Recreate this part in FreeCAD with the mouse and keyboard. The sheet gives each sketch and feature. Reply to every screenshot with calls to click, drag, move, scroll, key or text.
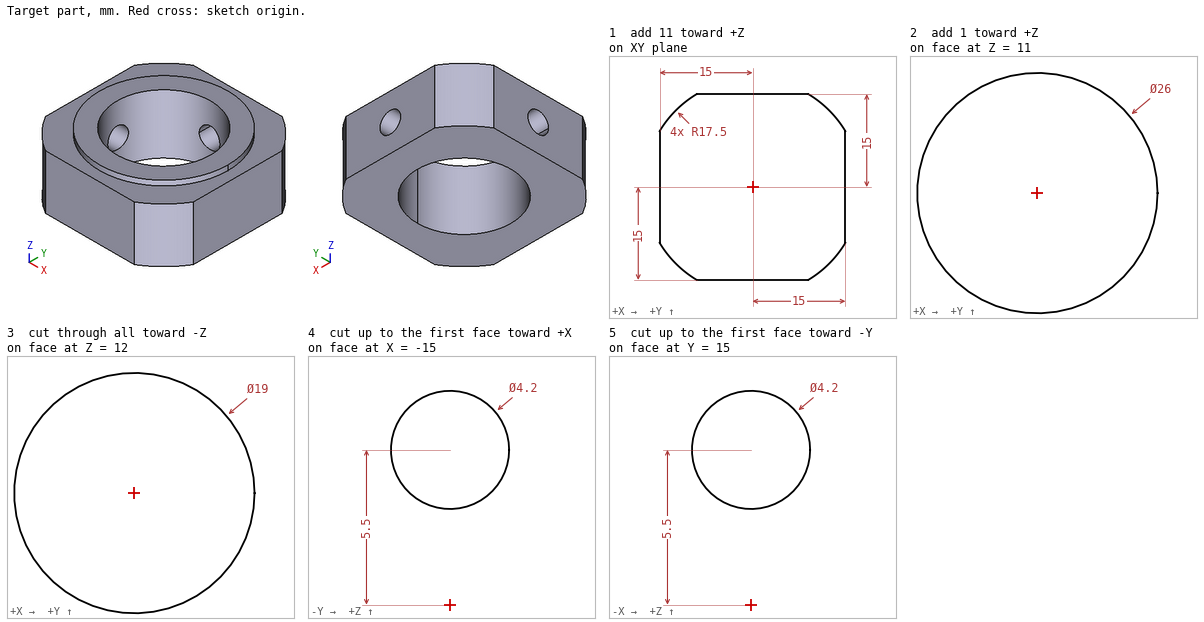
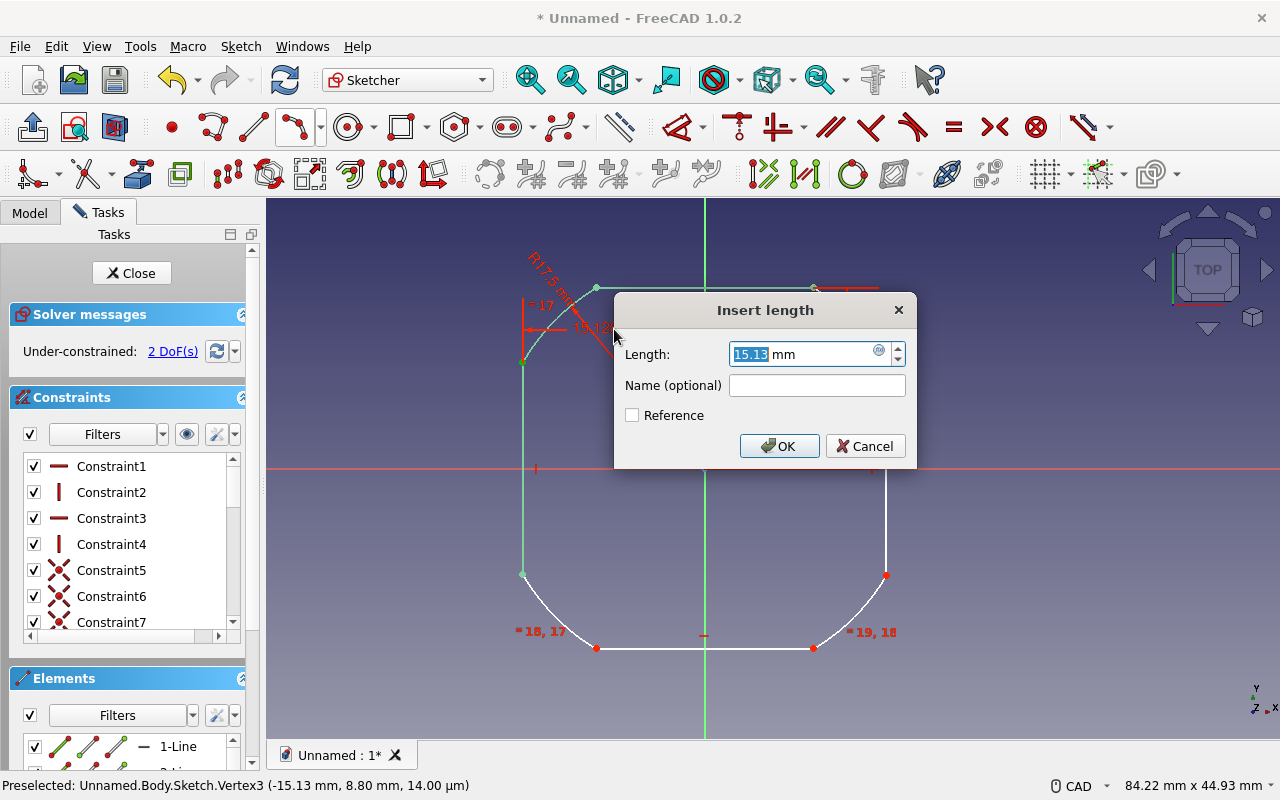
text(15)
key(Return)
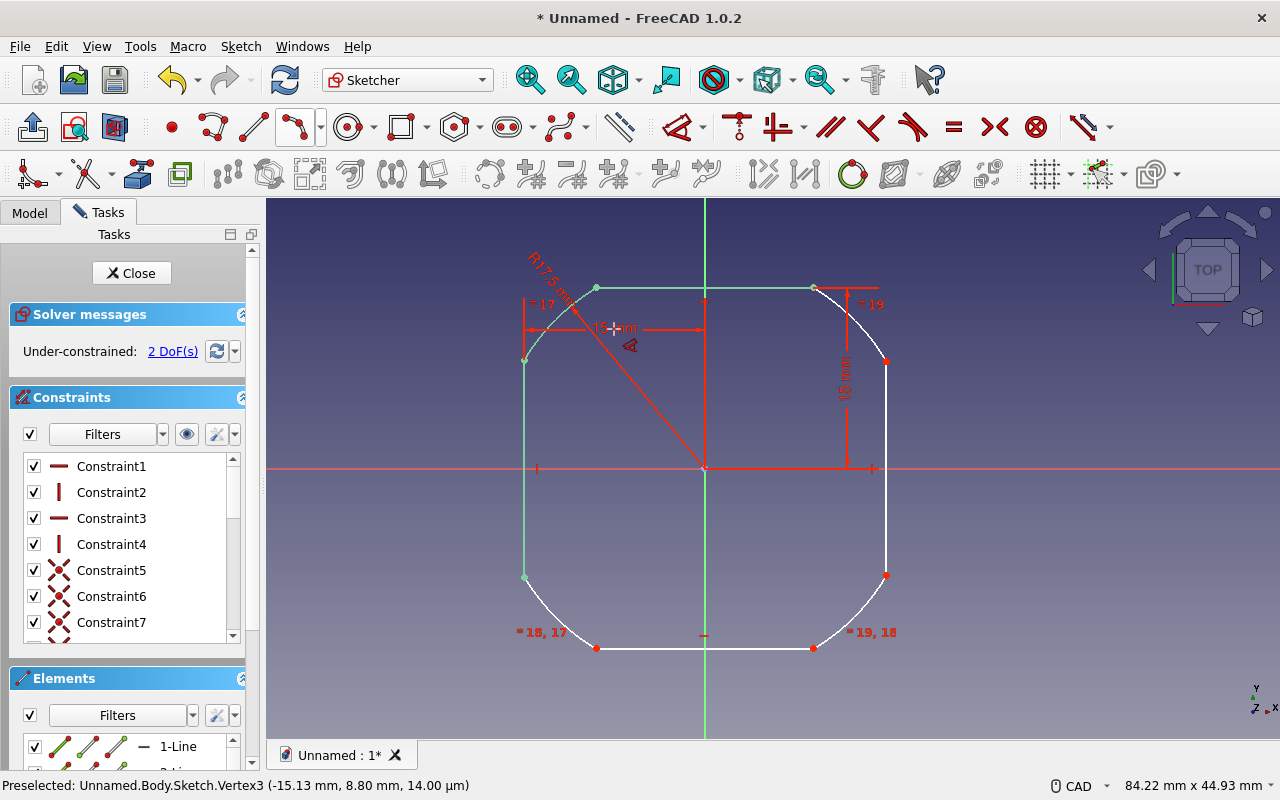
click(596, 649)
click(562, 559)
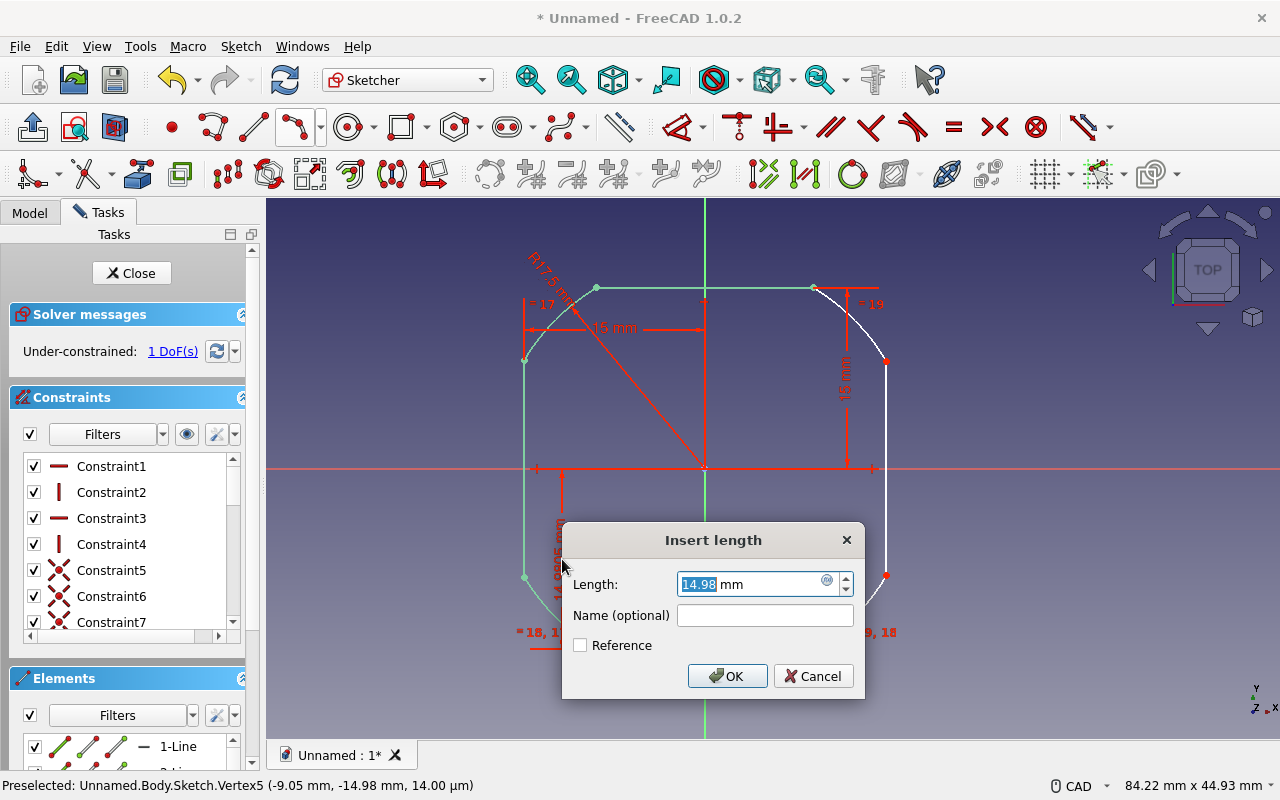
text(15)
key(Return)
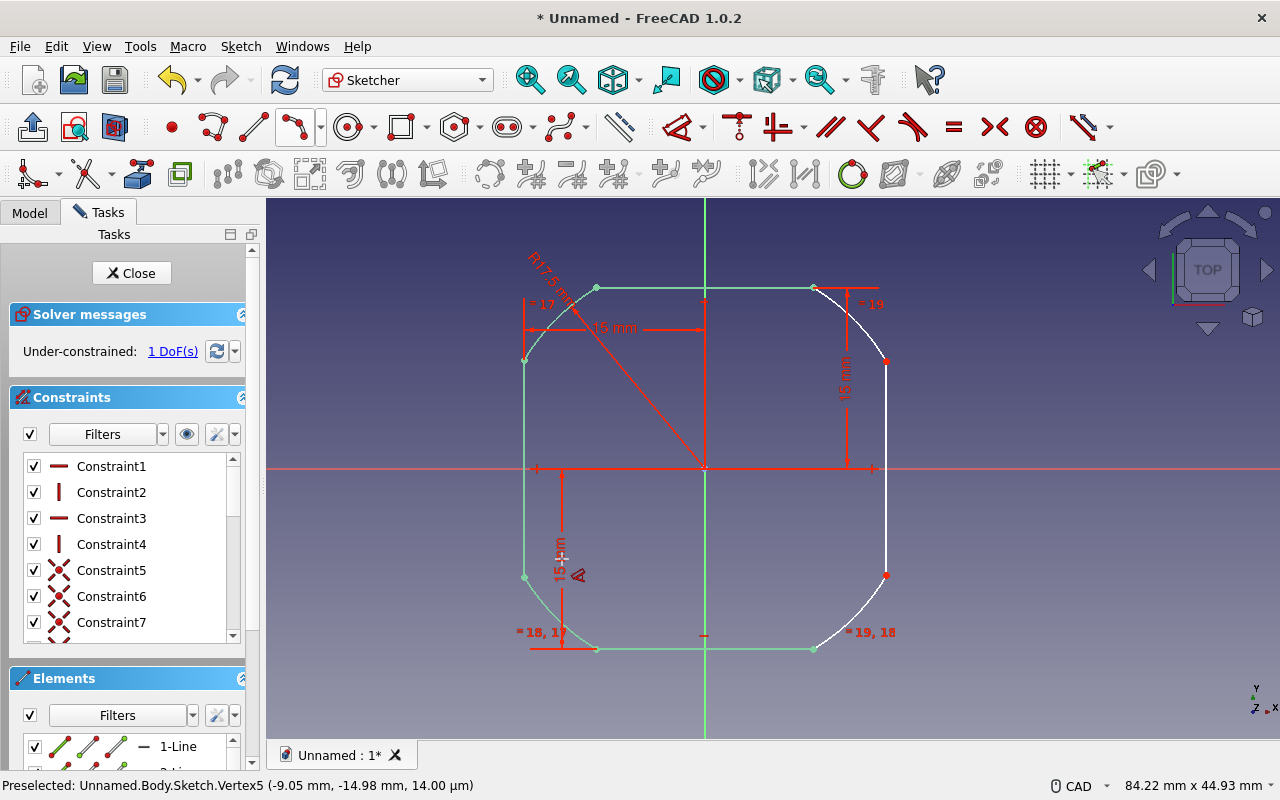
click(886, 576)
click(796, 610)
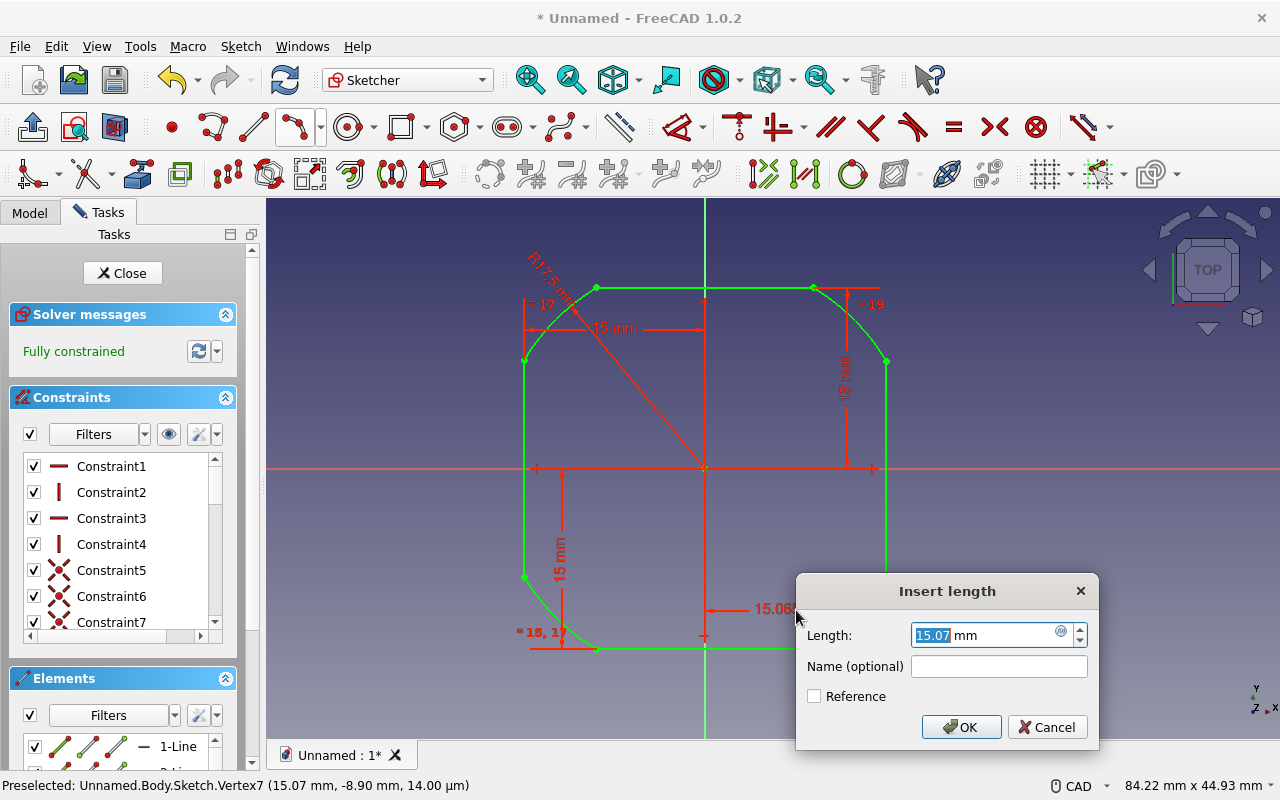
text(15)
key(Return)
key(Escape)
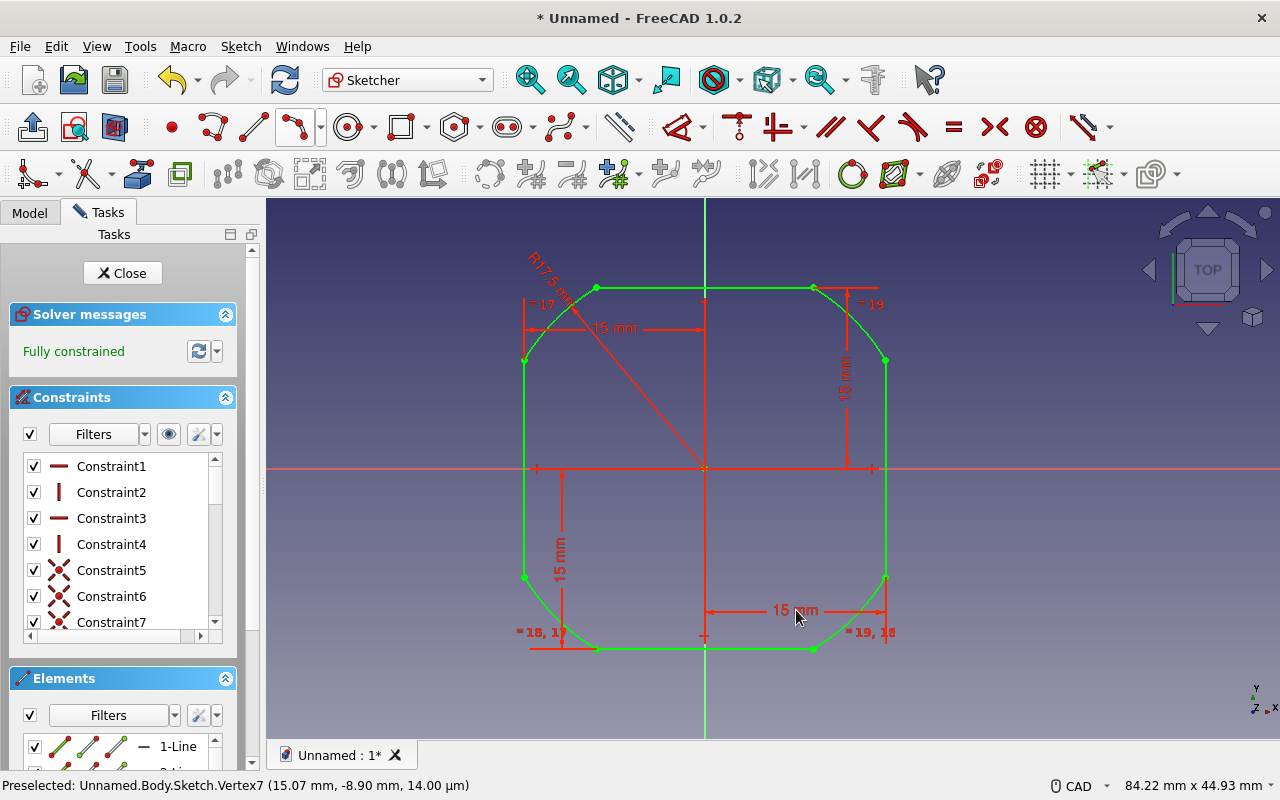
click(123, 273)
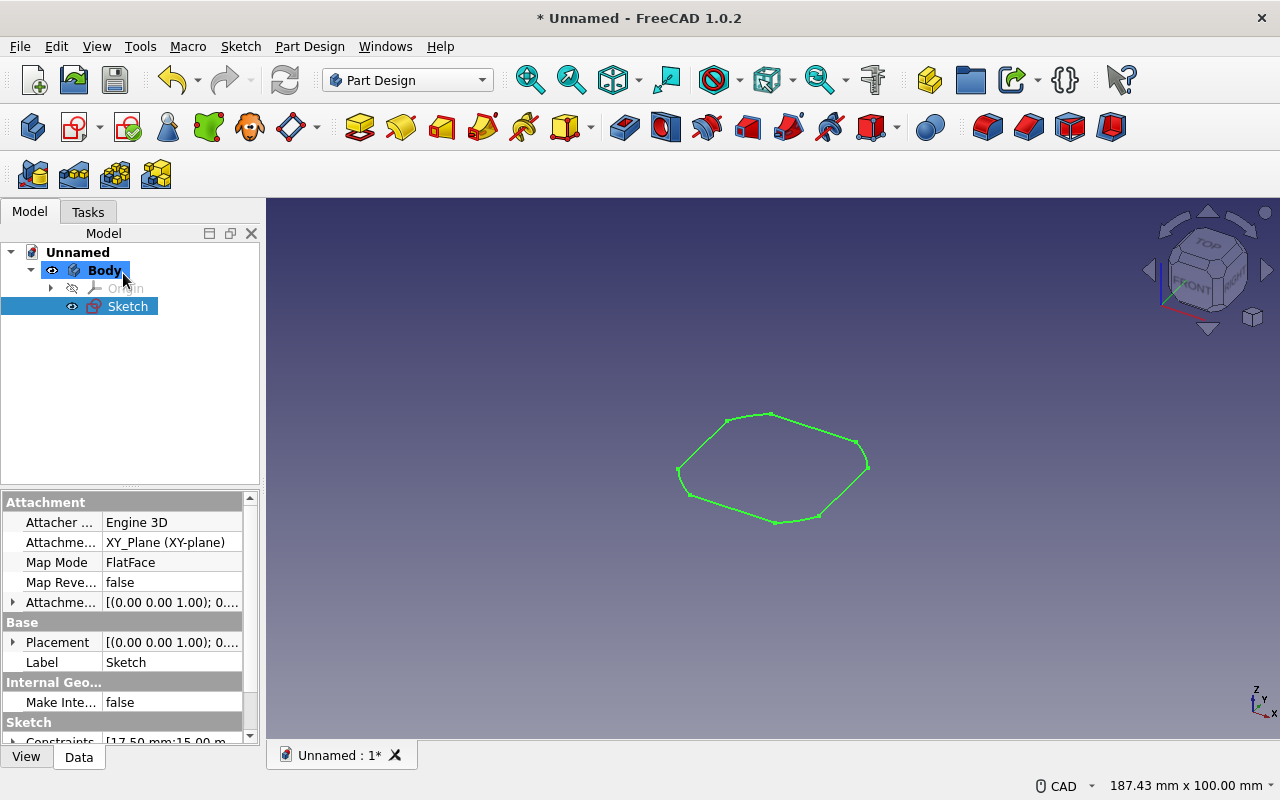
click(360, 128)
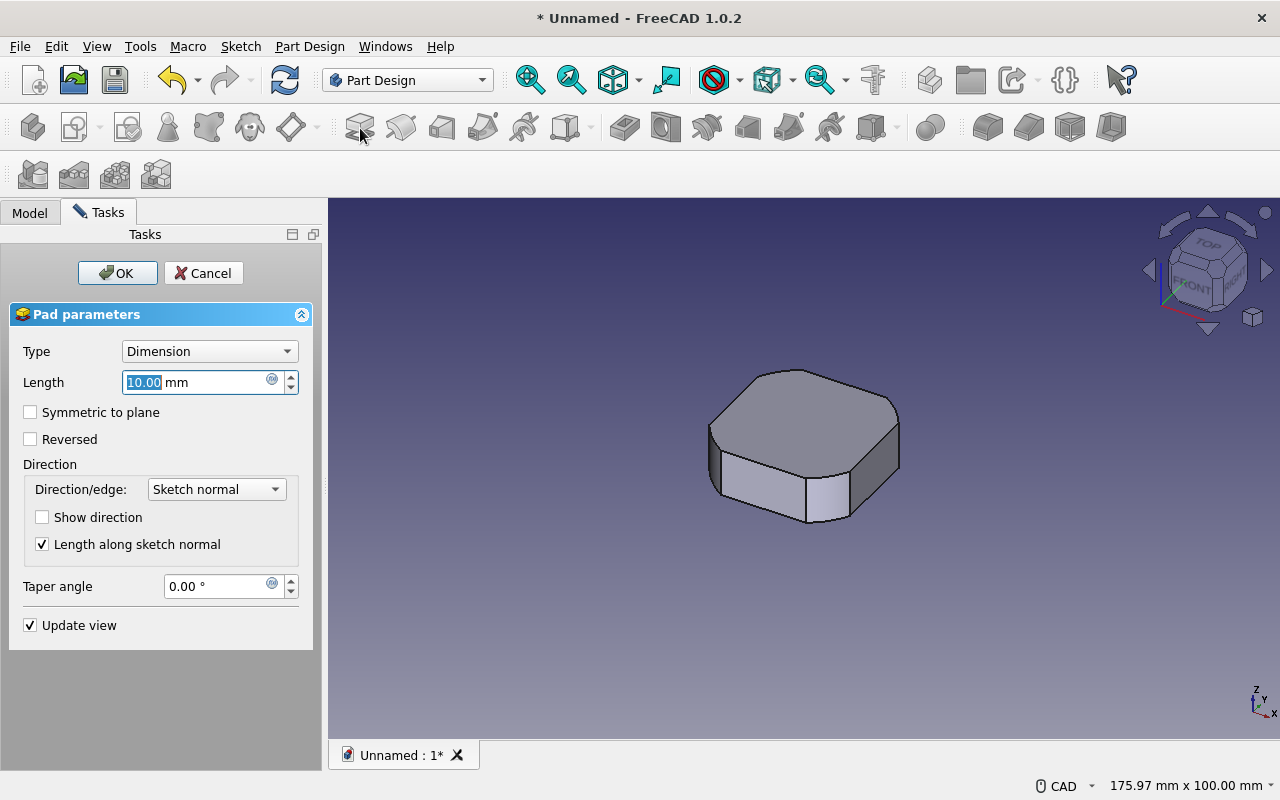
text(11)
key(Tab)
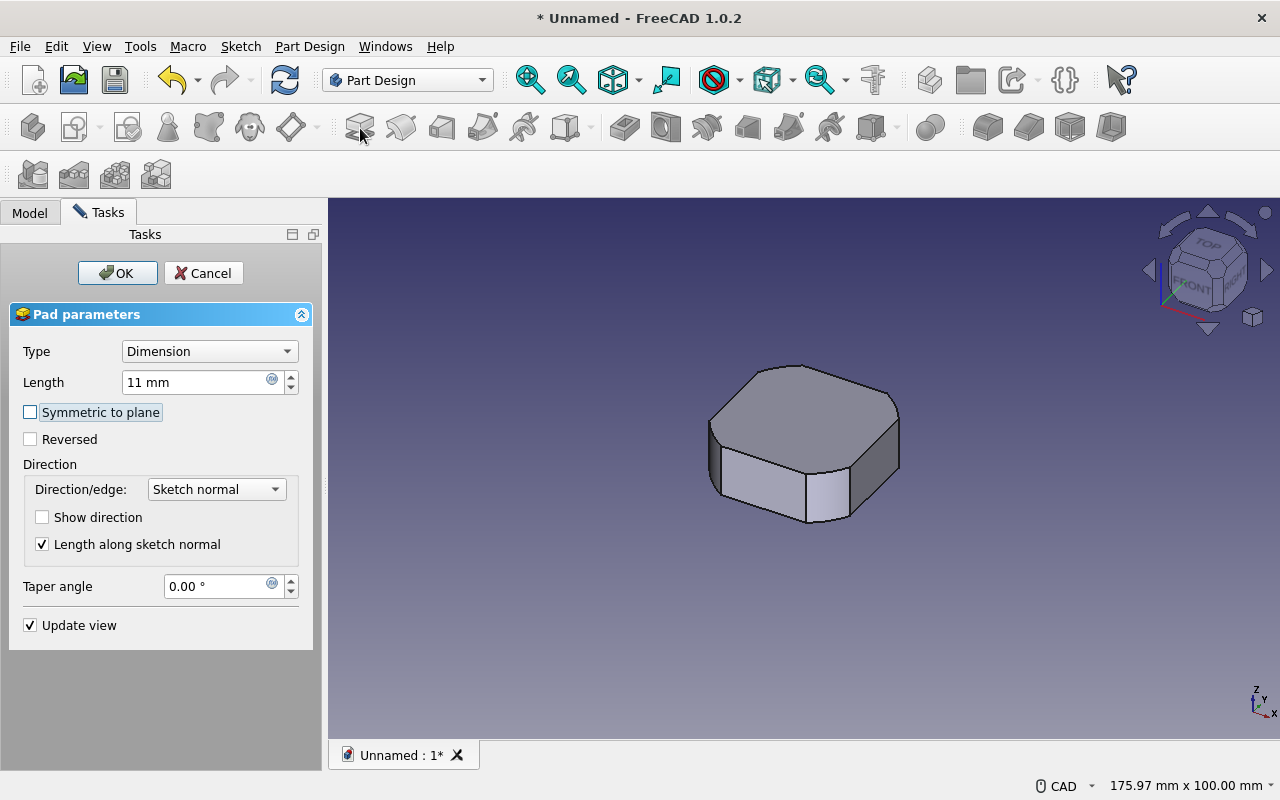
click(118, 273)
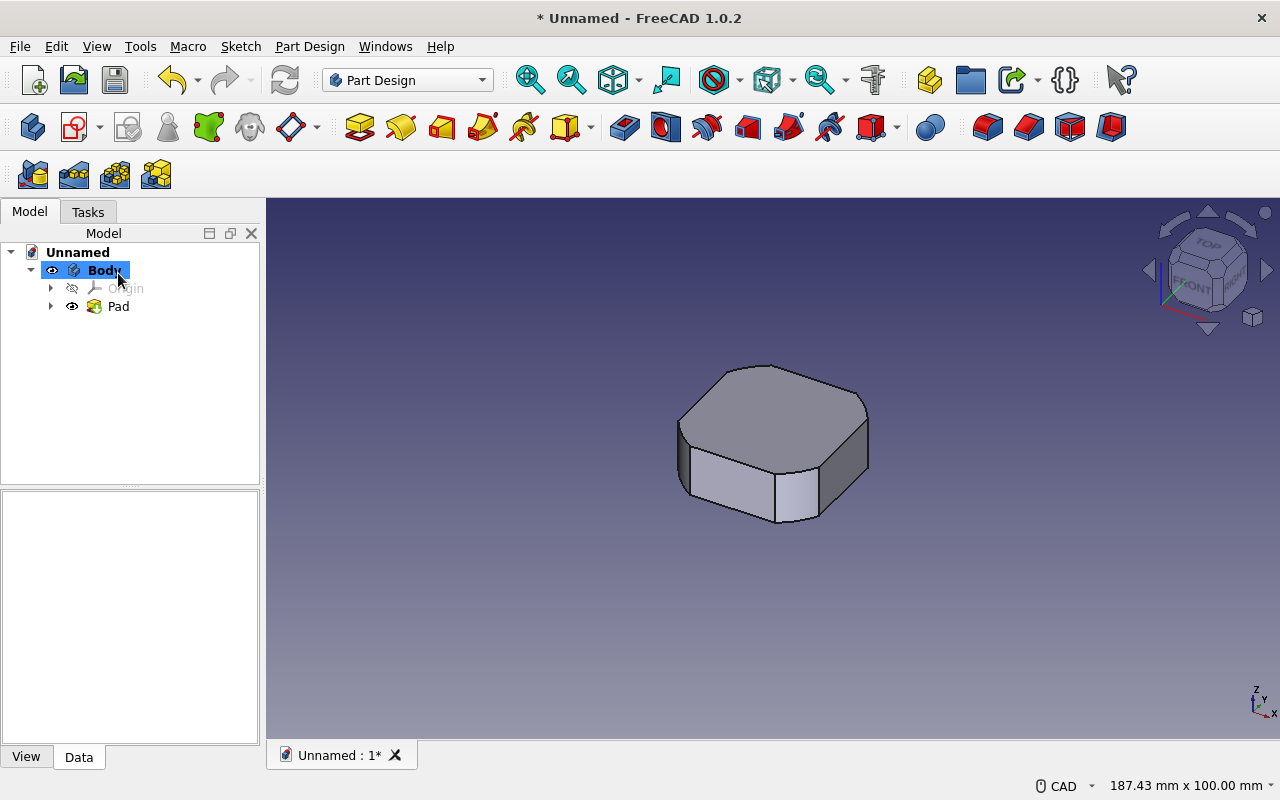
click(531, 80)